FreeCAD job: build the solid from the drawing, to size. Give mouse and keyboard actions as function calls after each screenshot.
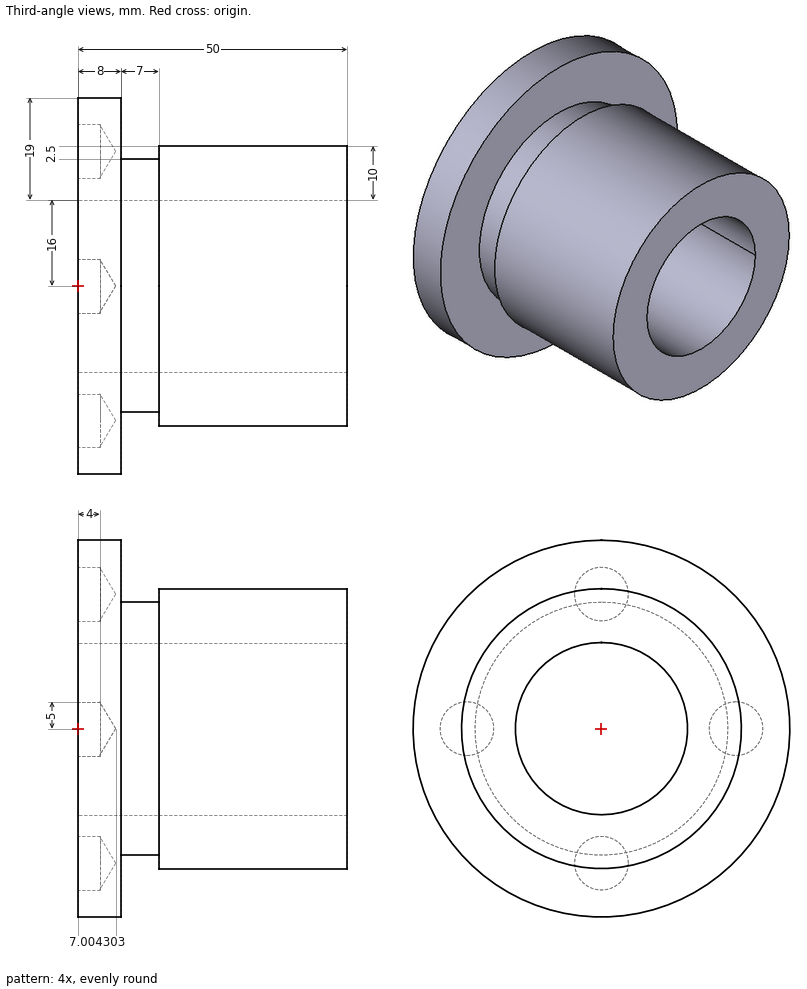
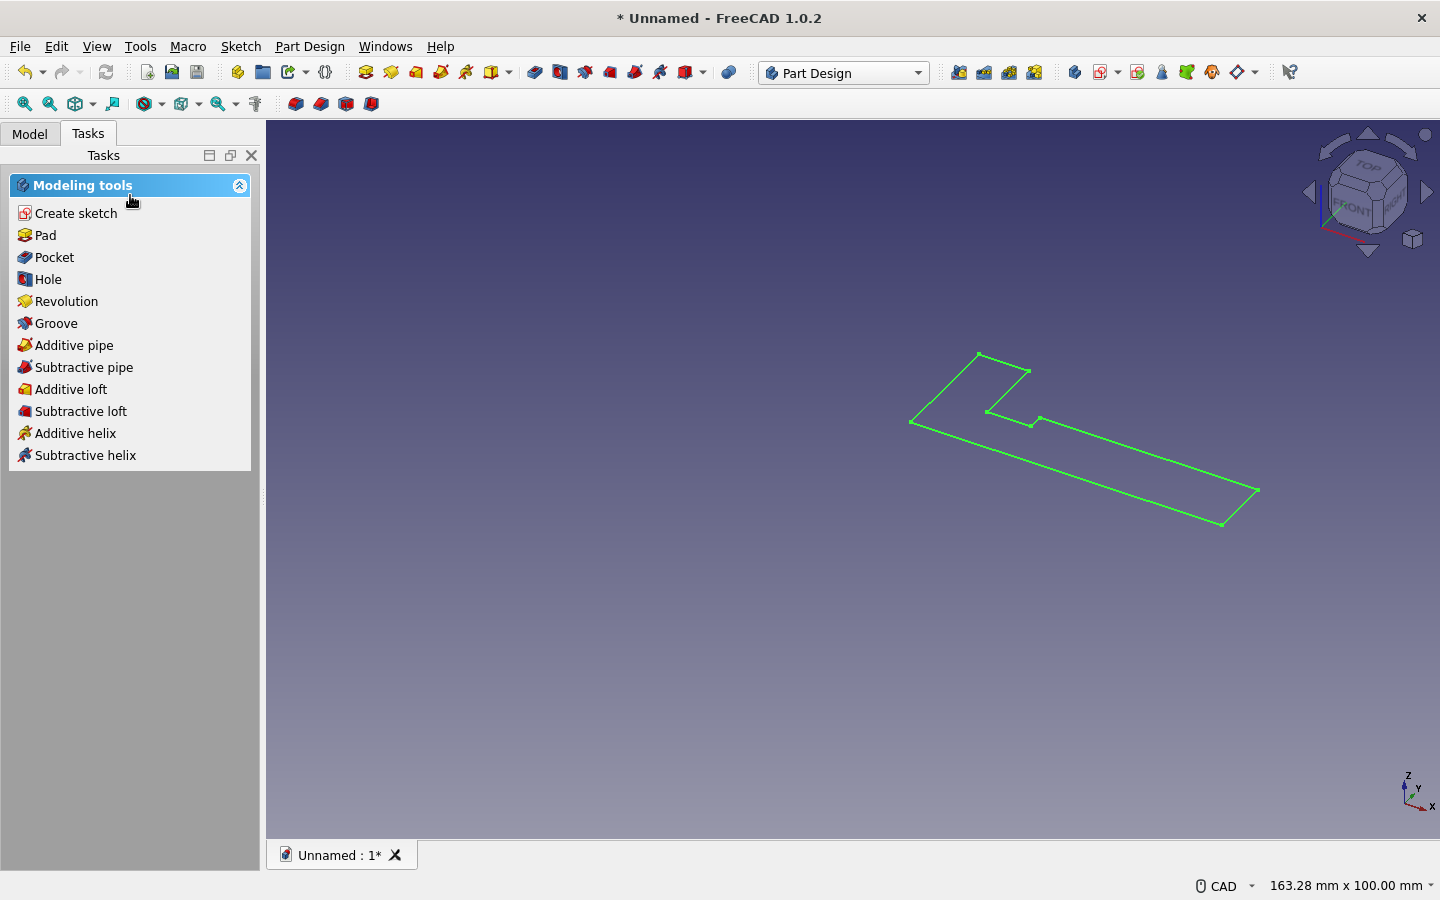
click(391, 72)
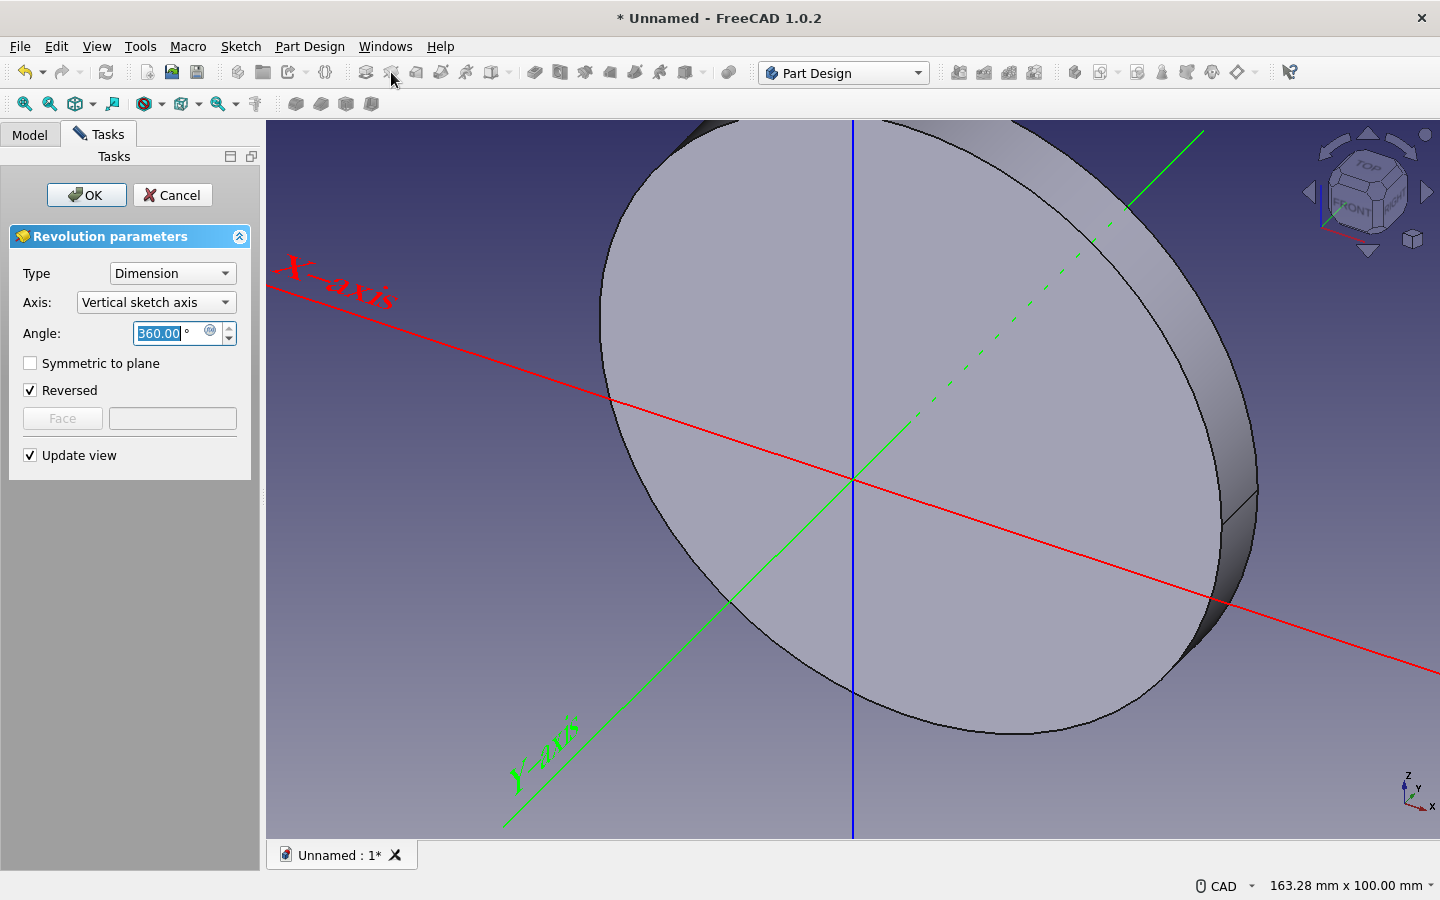
click(157, 302)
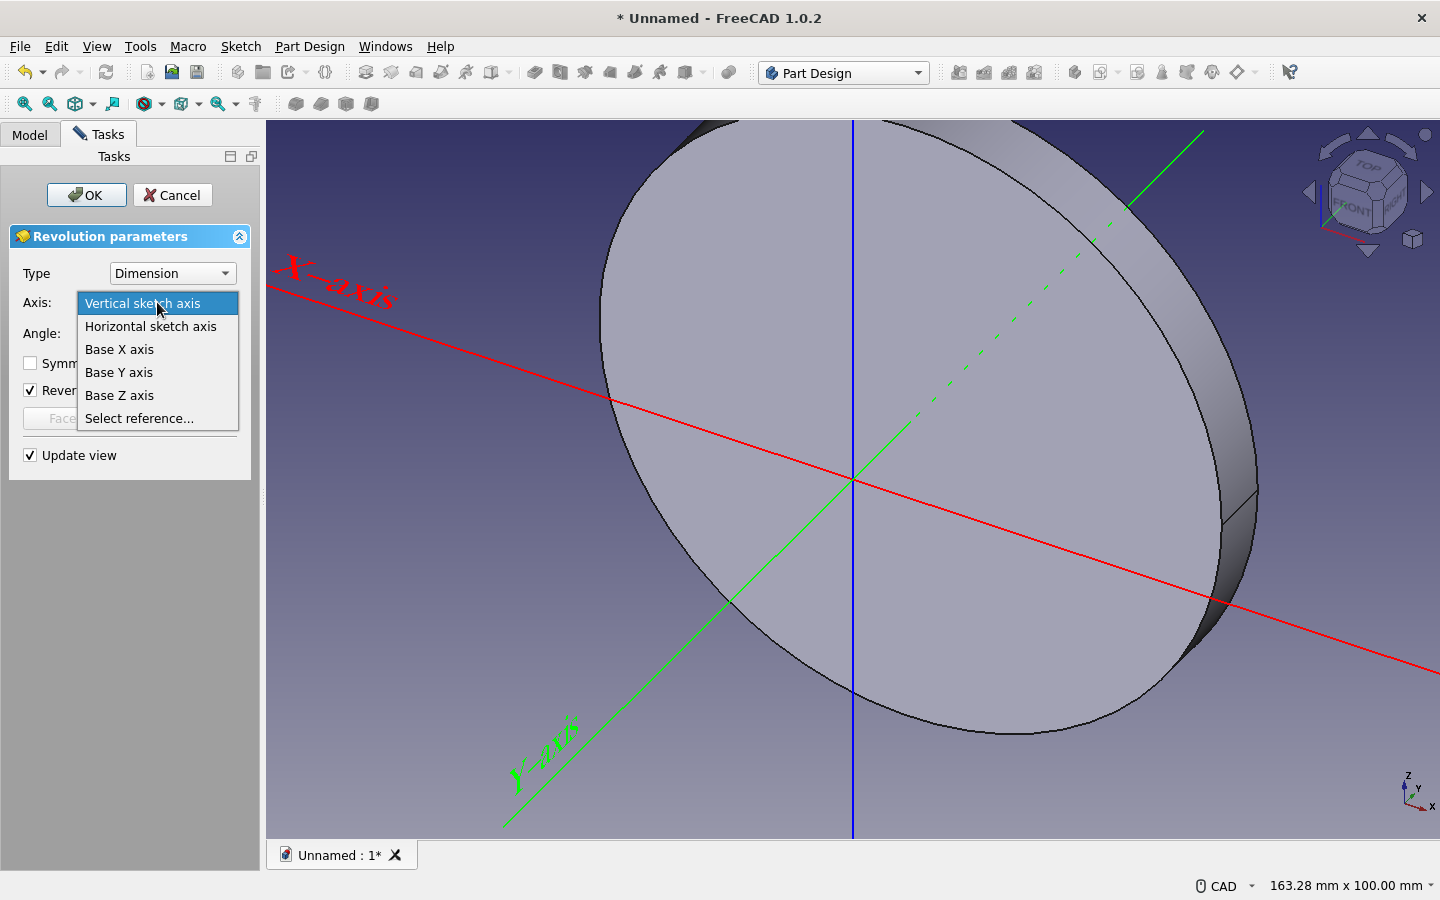
click(156, 326)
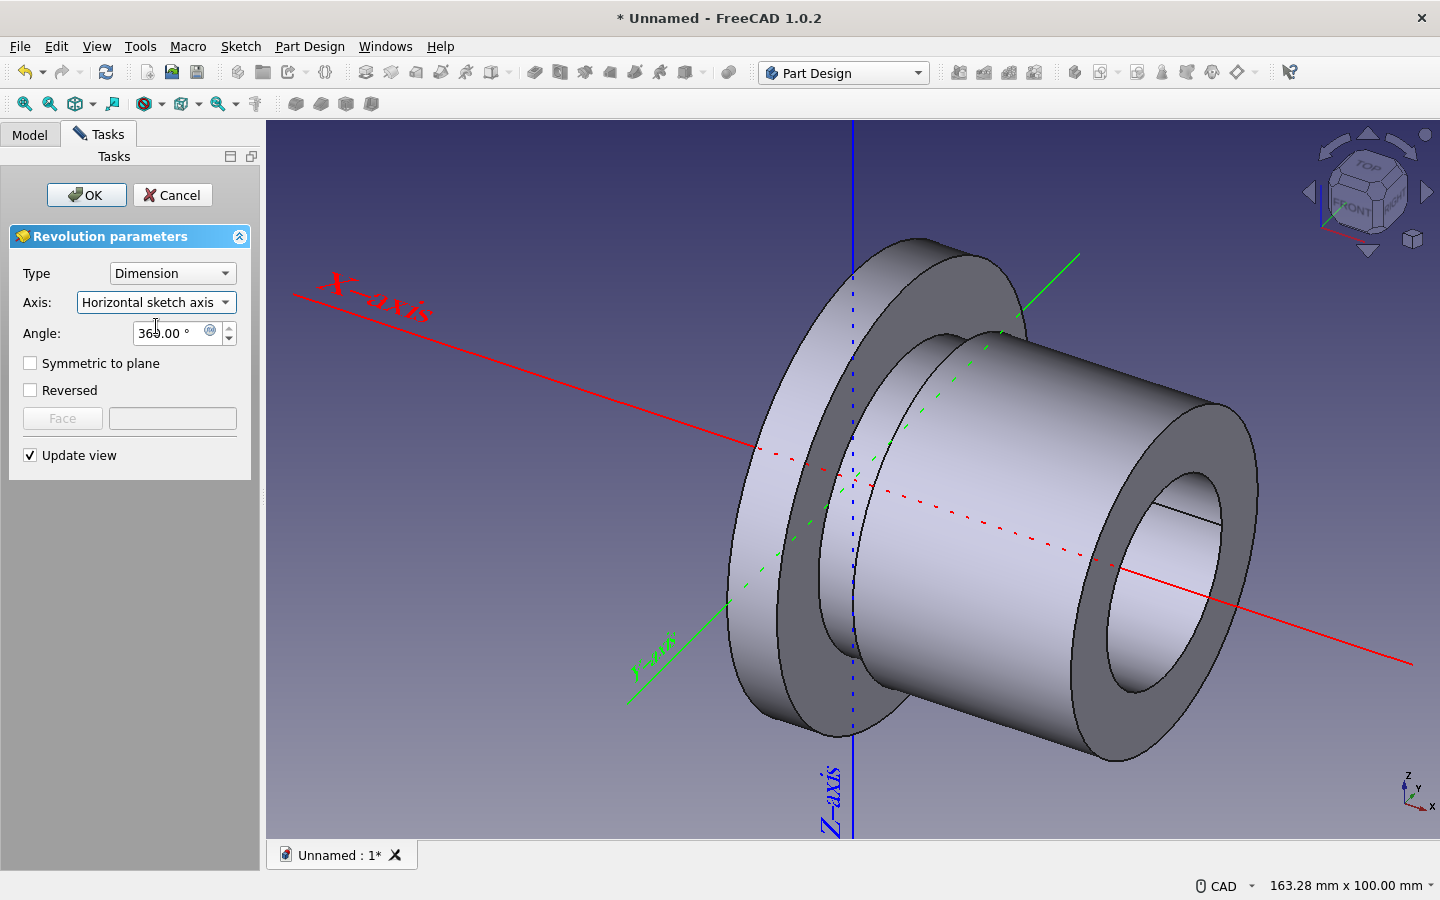
click(87, 195)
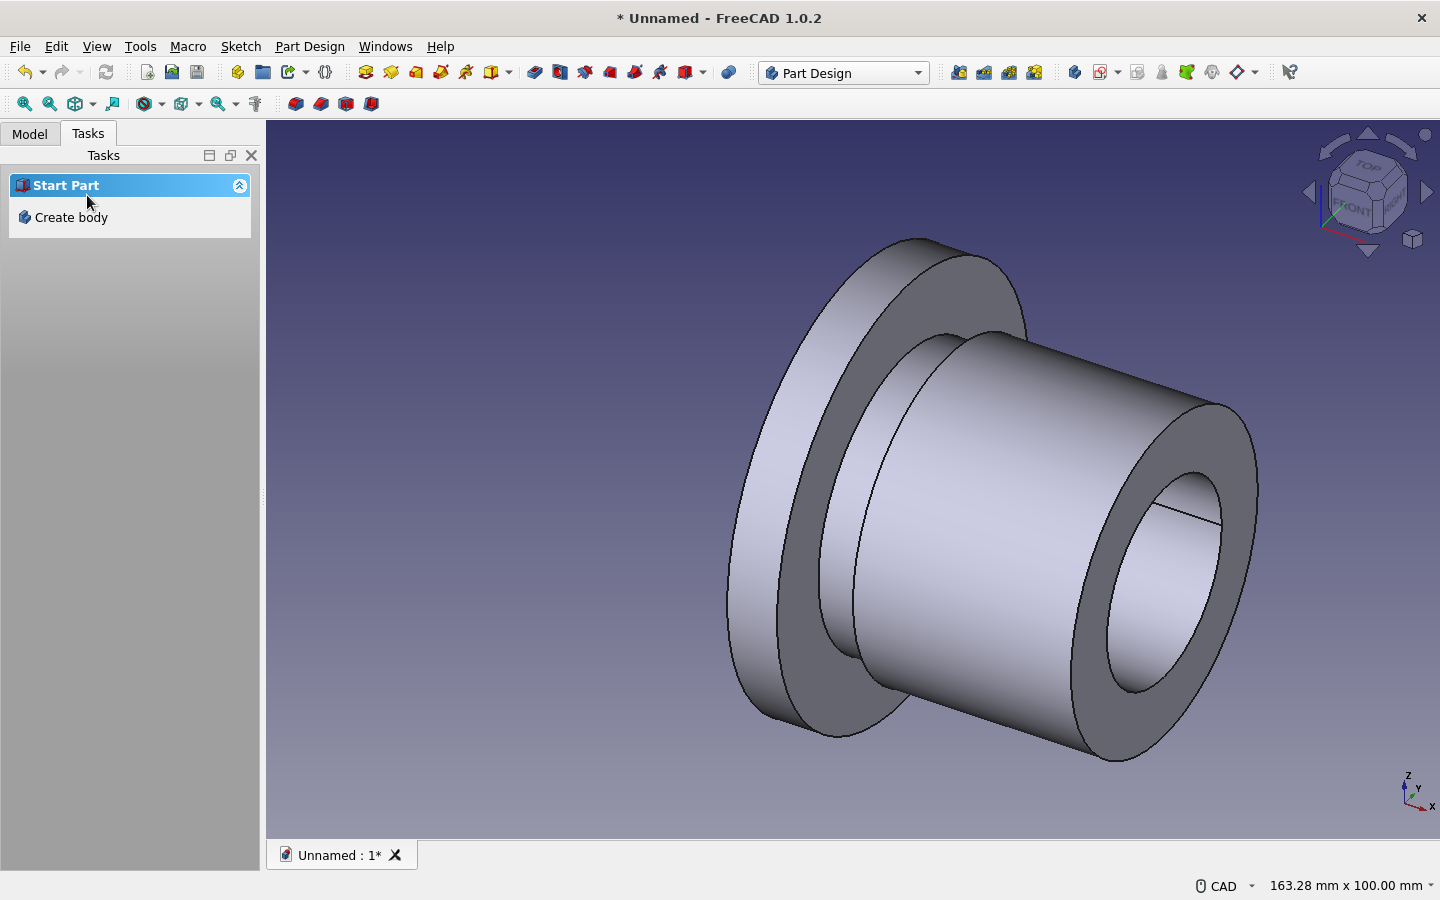
click(25, 104)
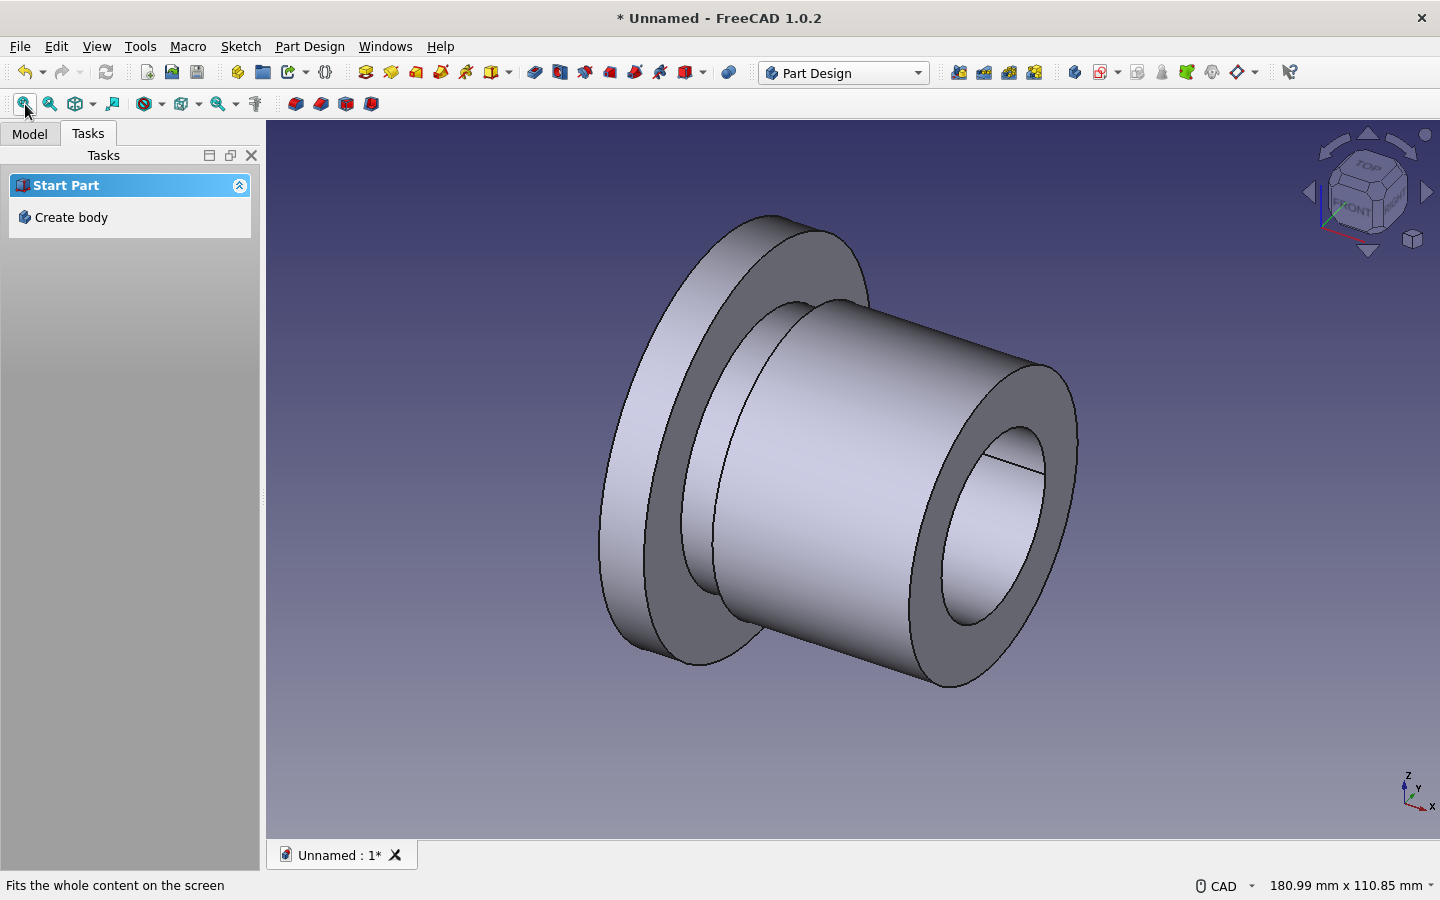
click(30, 134)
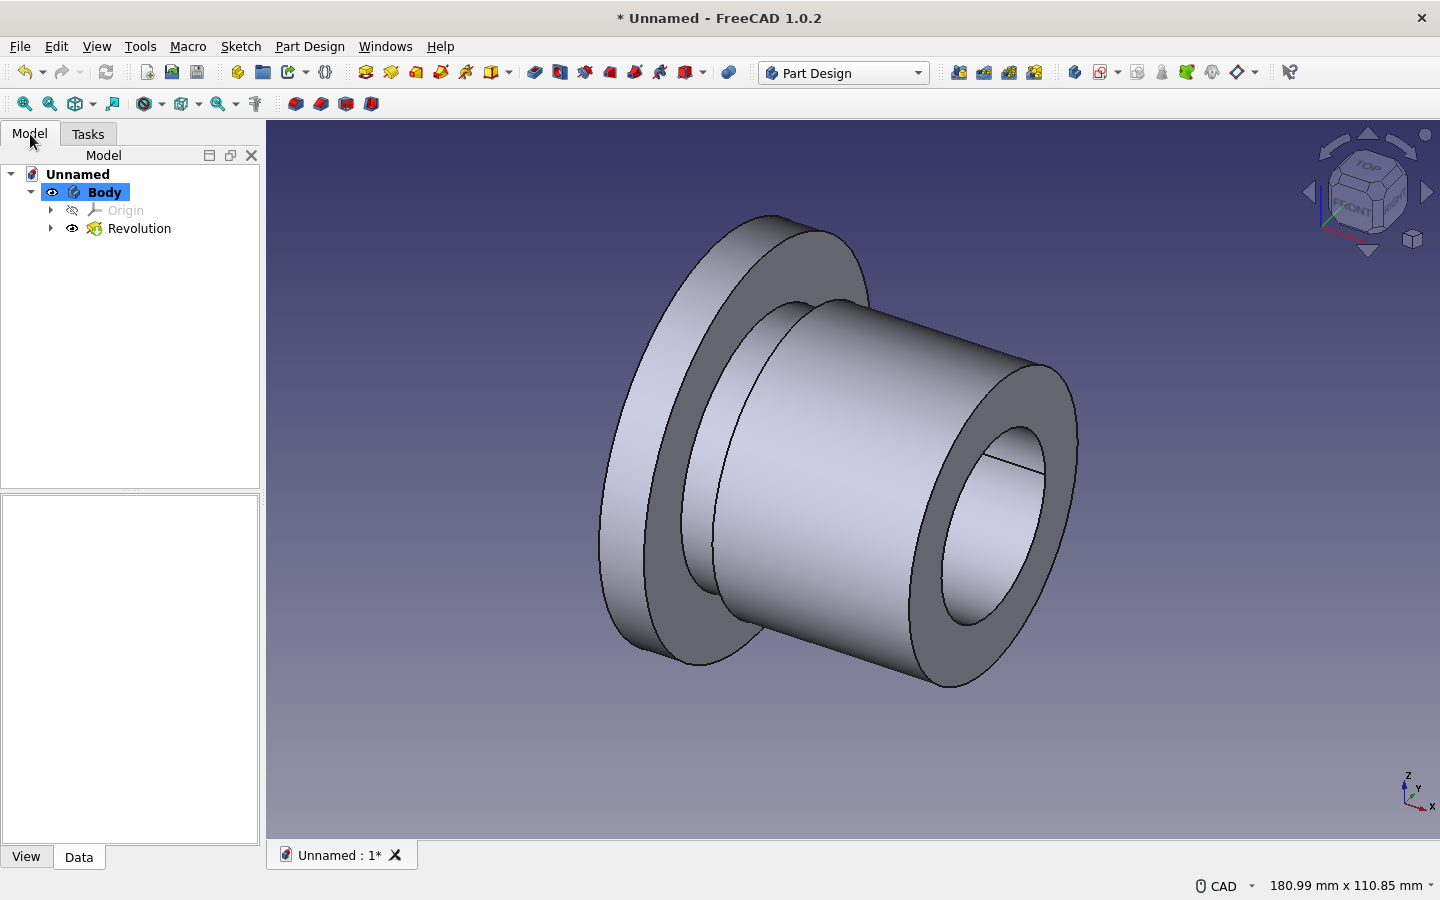
click(51, 210)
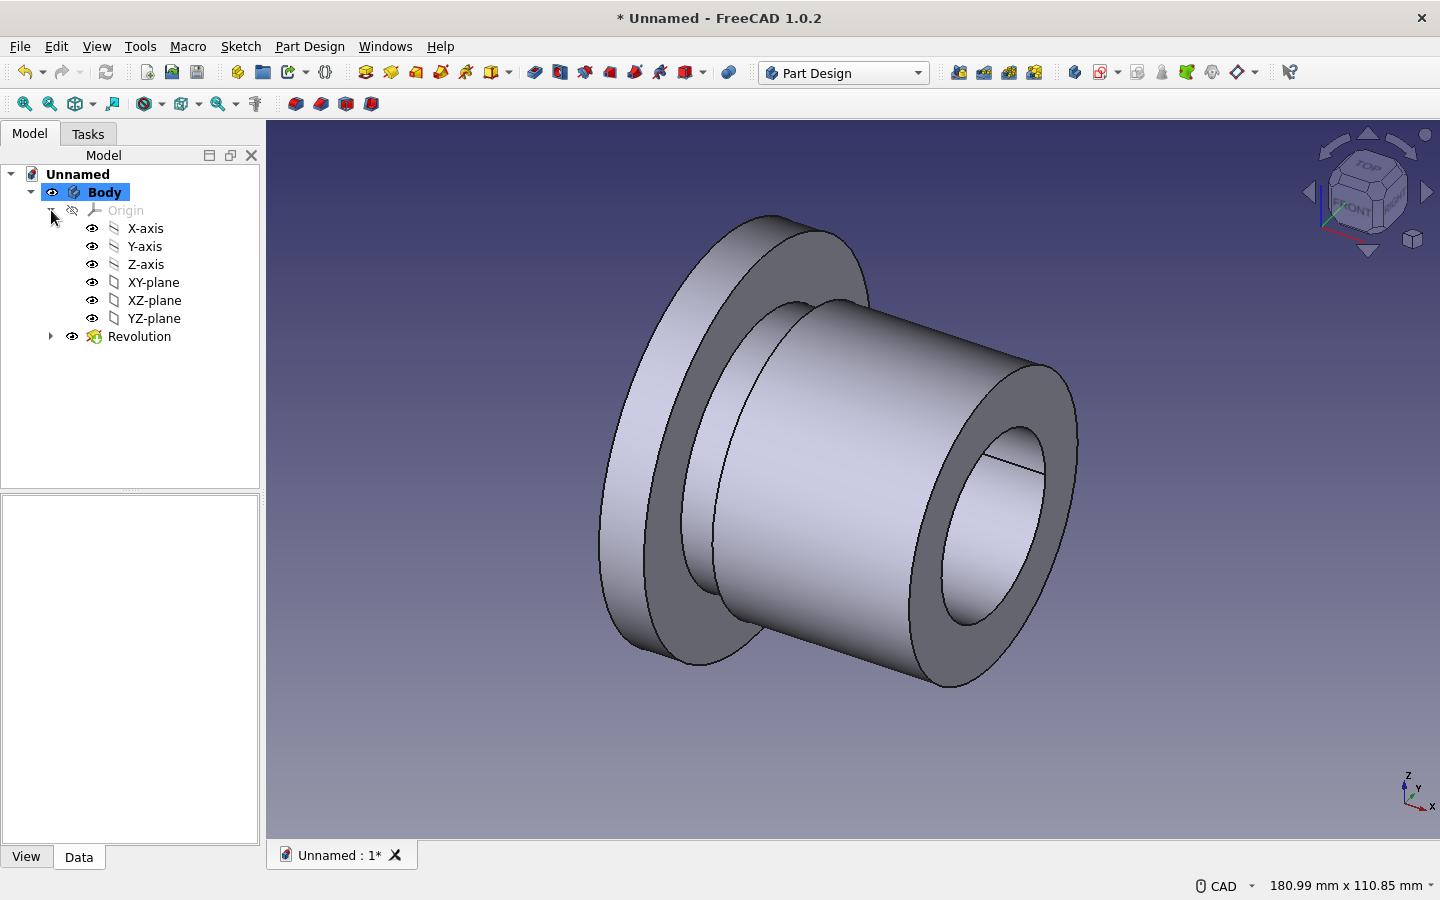
click(137, 300)